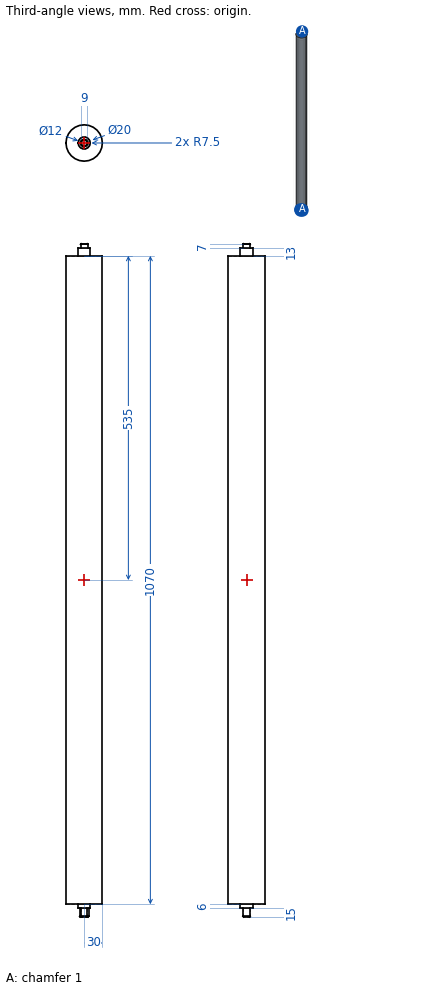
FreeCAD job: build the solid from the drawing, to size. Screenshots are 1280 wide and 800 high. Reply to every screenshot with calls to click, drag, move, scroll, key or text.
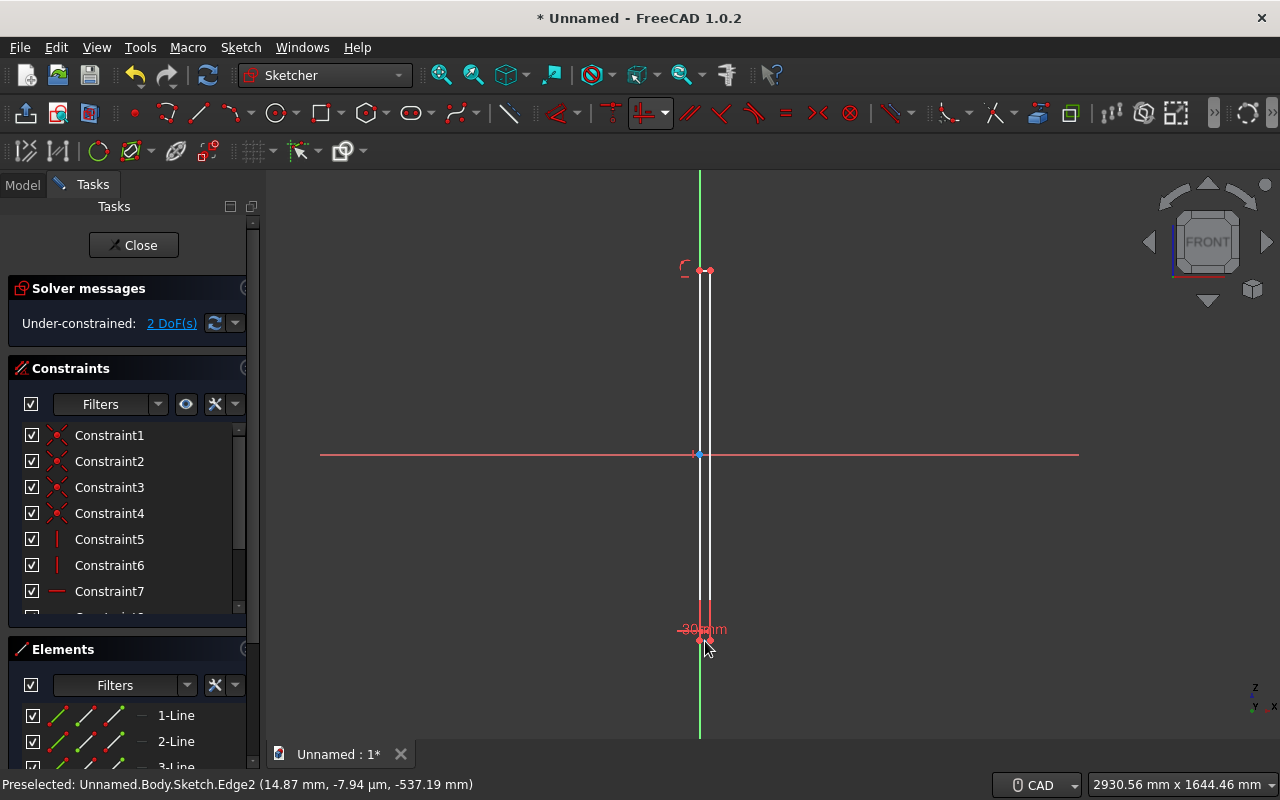
scroll(700, 567, up, 2)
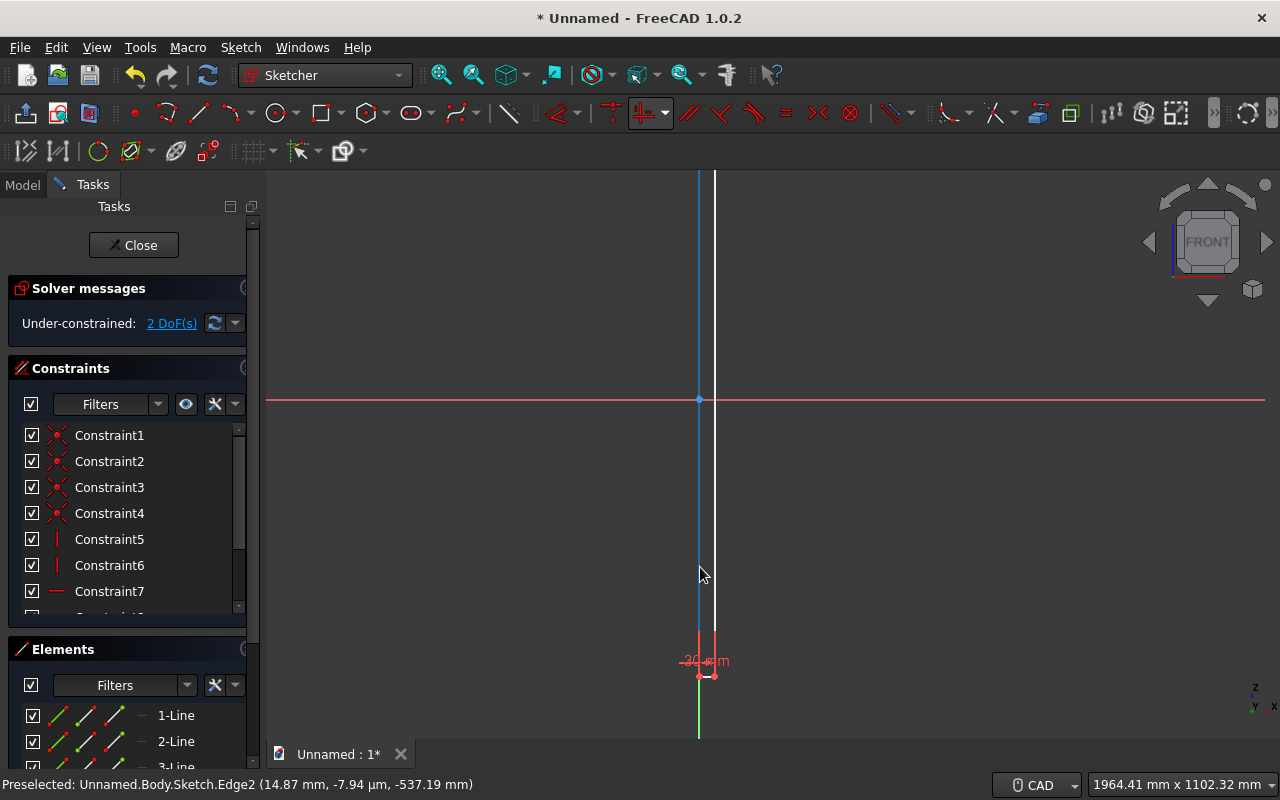
click(699, 566)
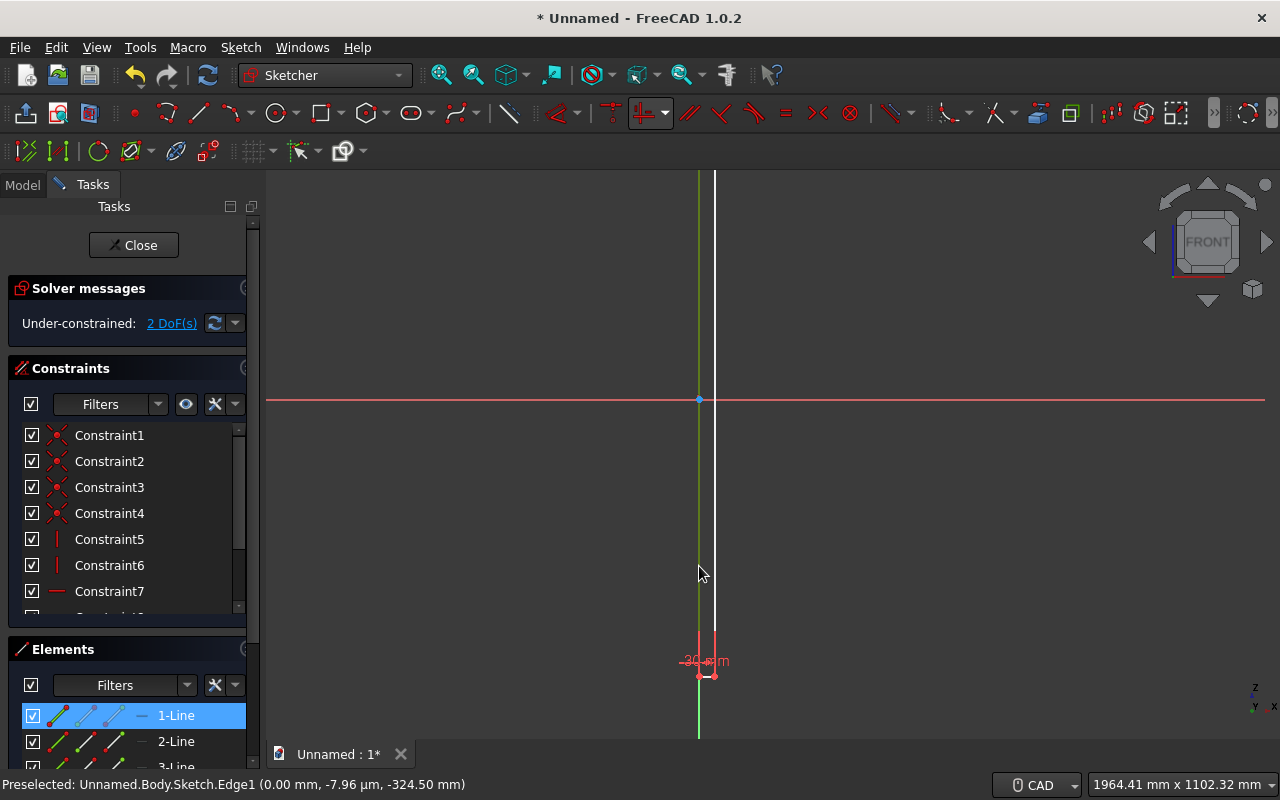
key(i)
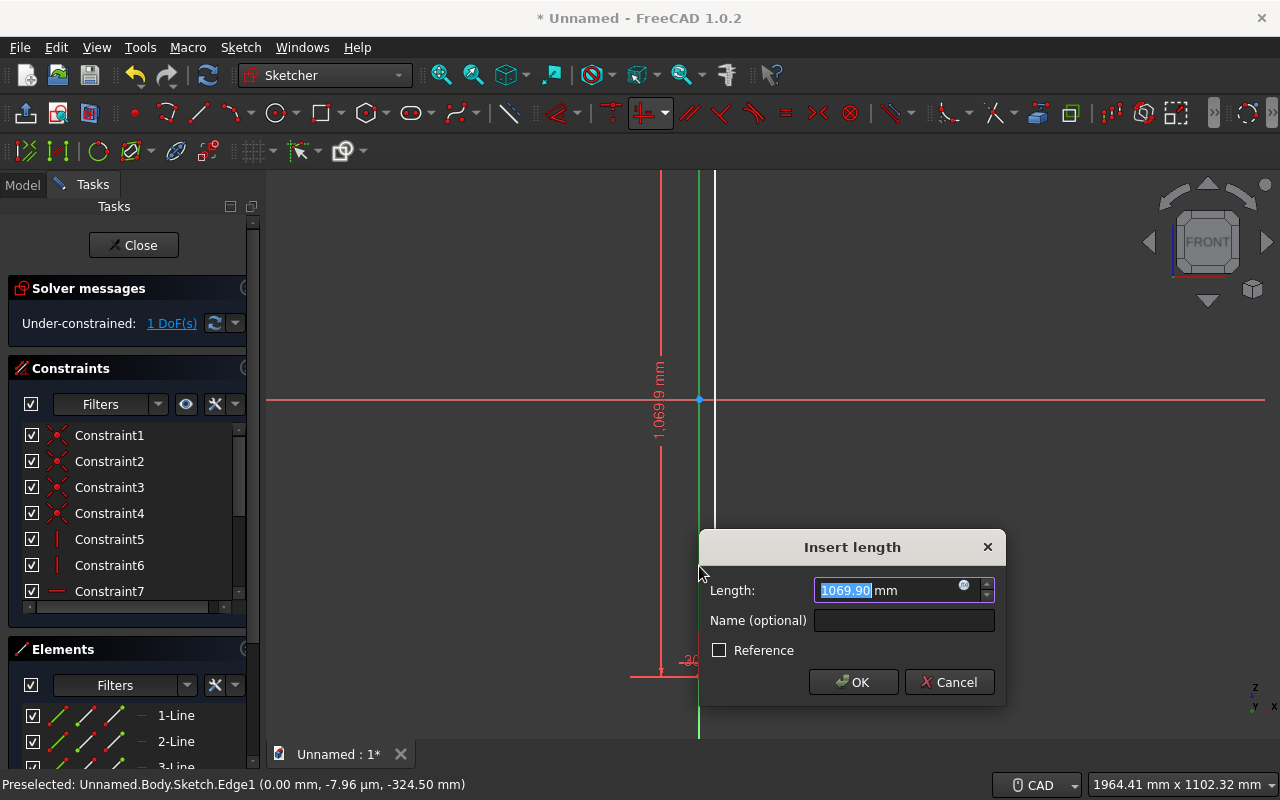
text(1070)
key(Return)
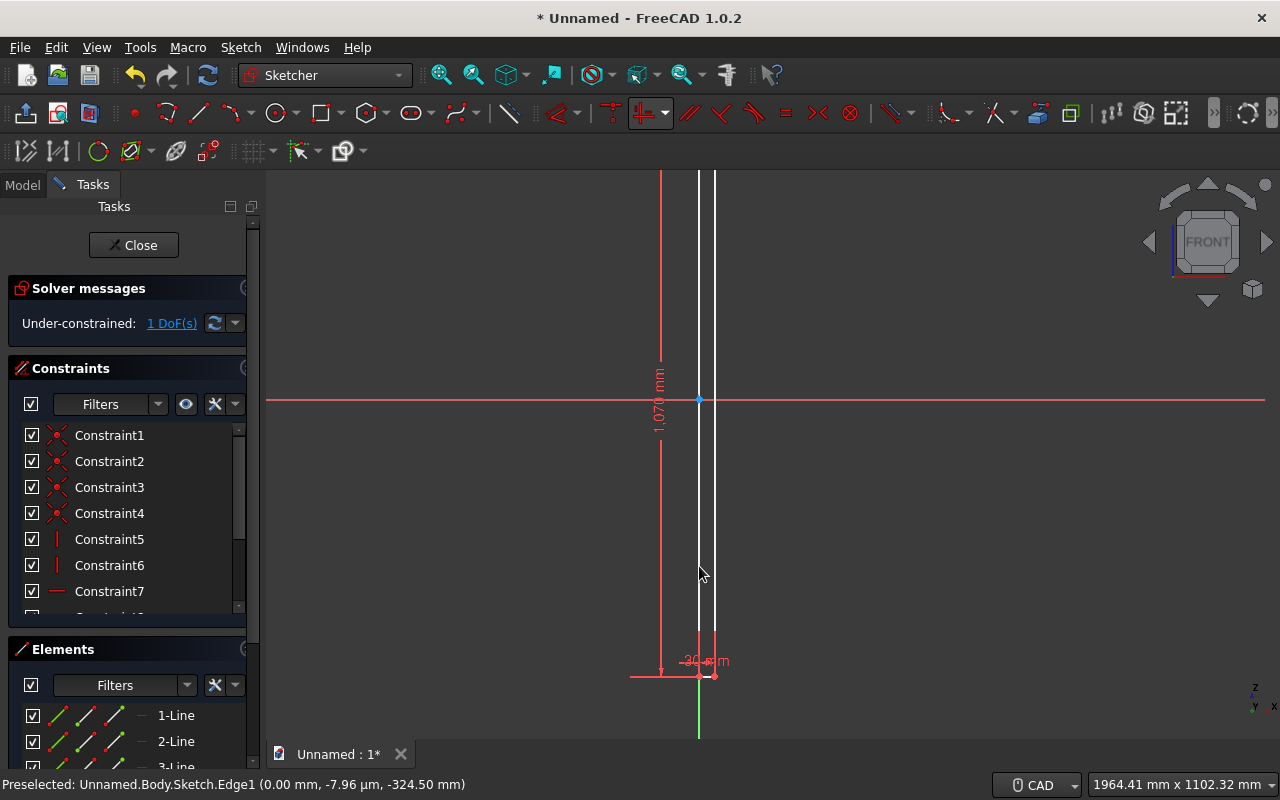
scroll(699, 566, down, 2)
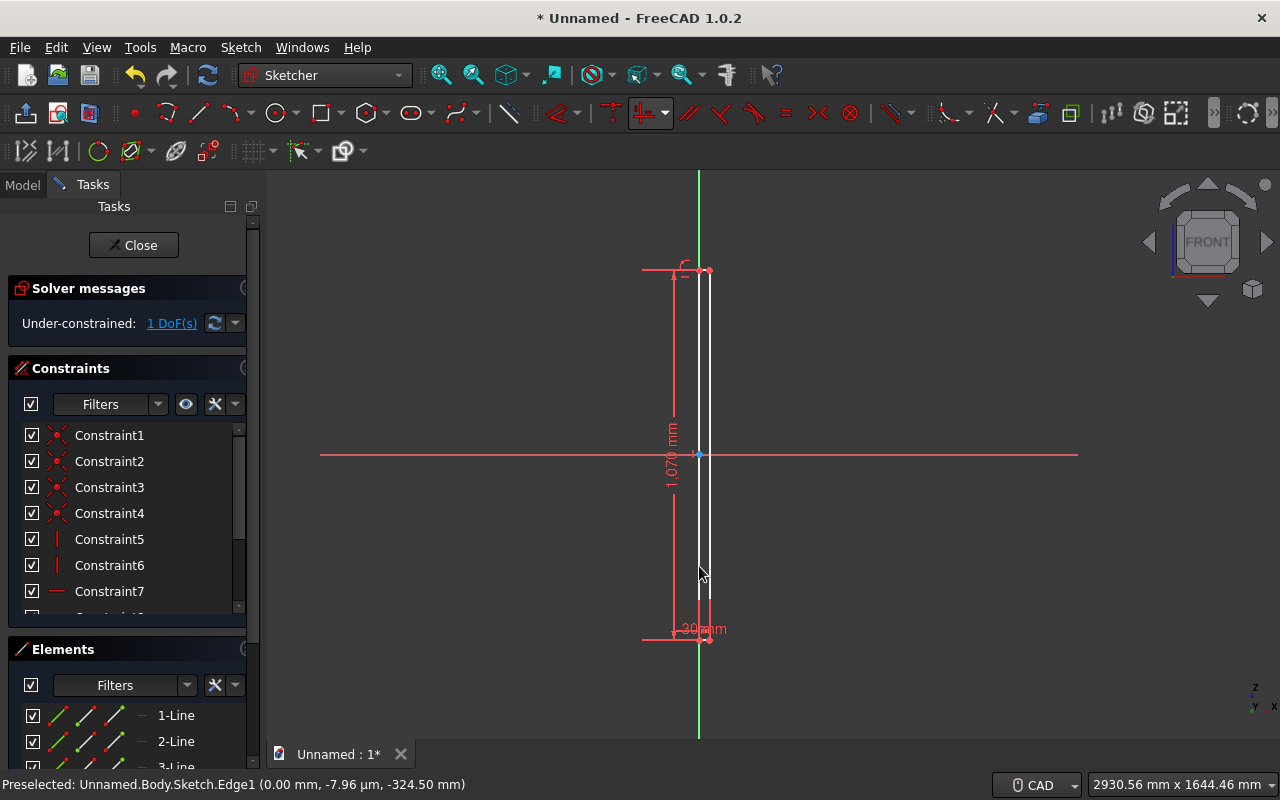
click(699, 270)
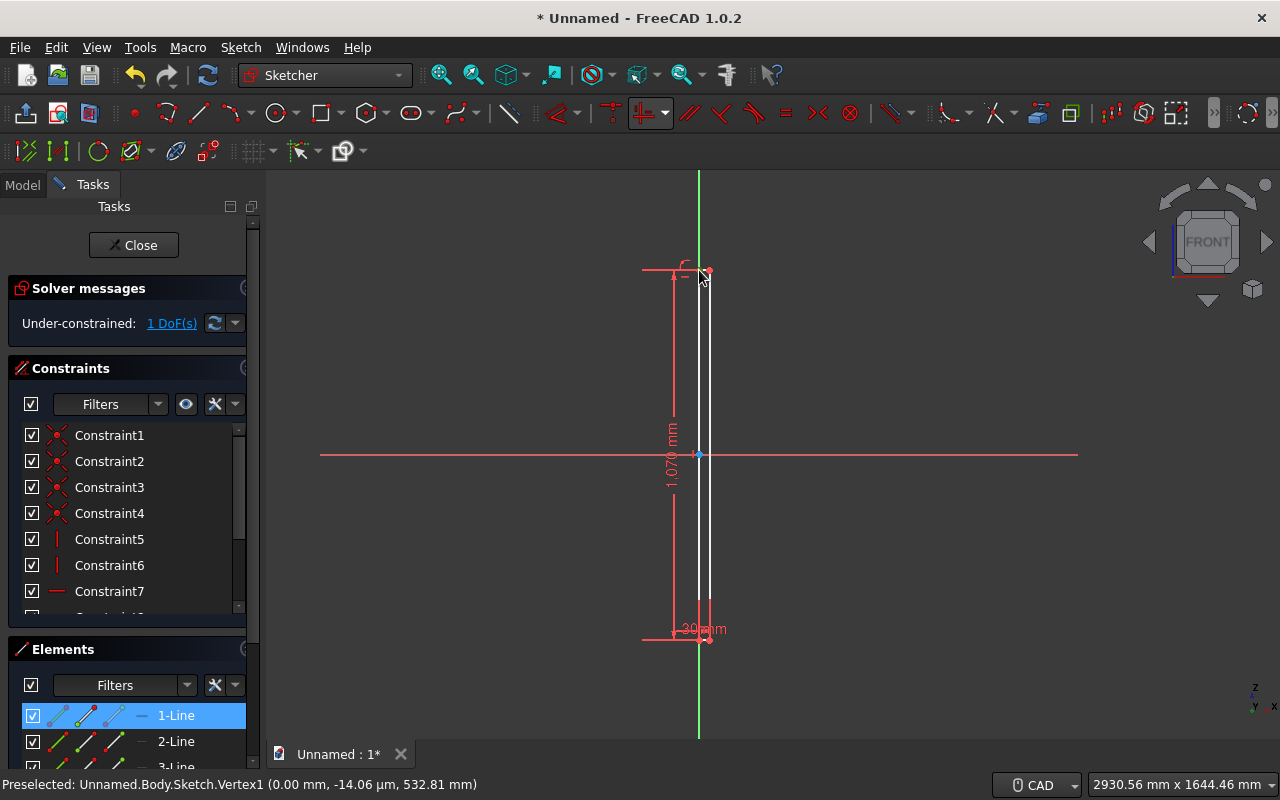
key(i)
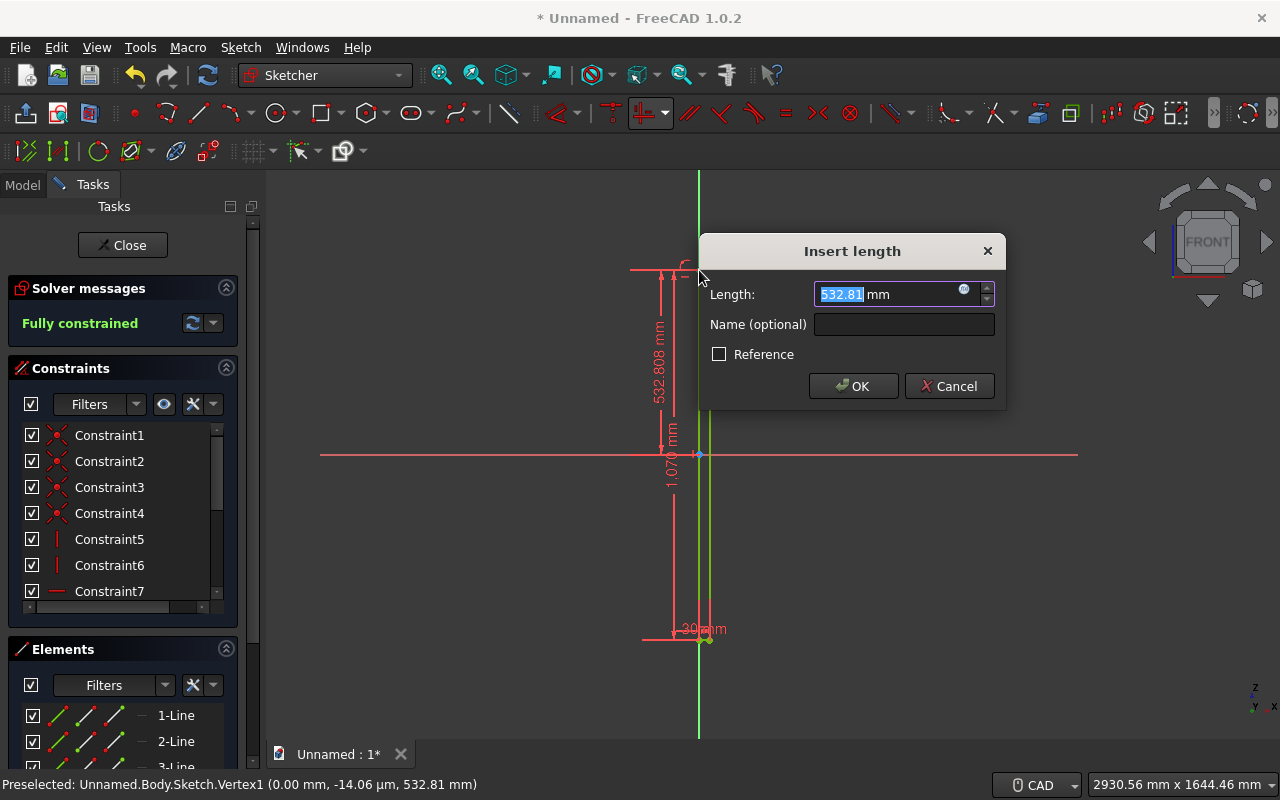
text(535)
key(Return)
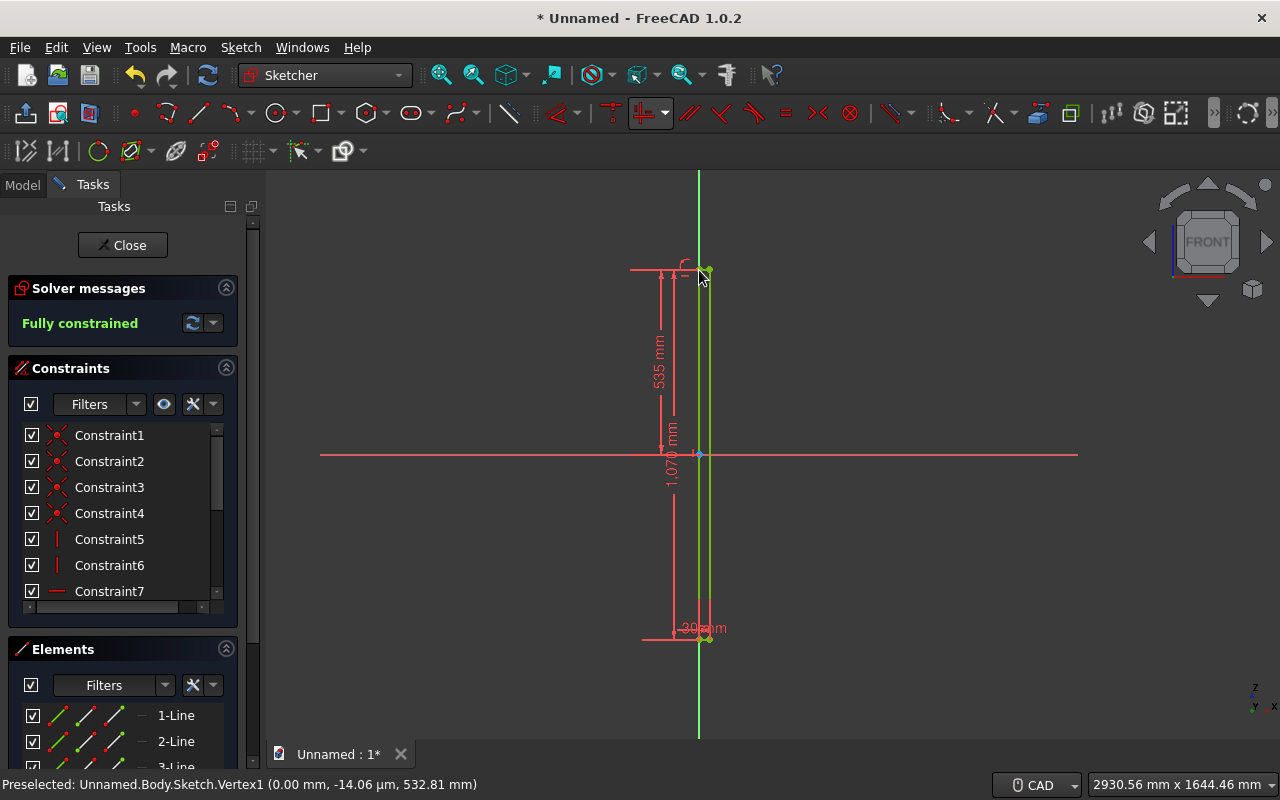
click(123, 245)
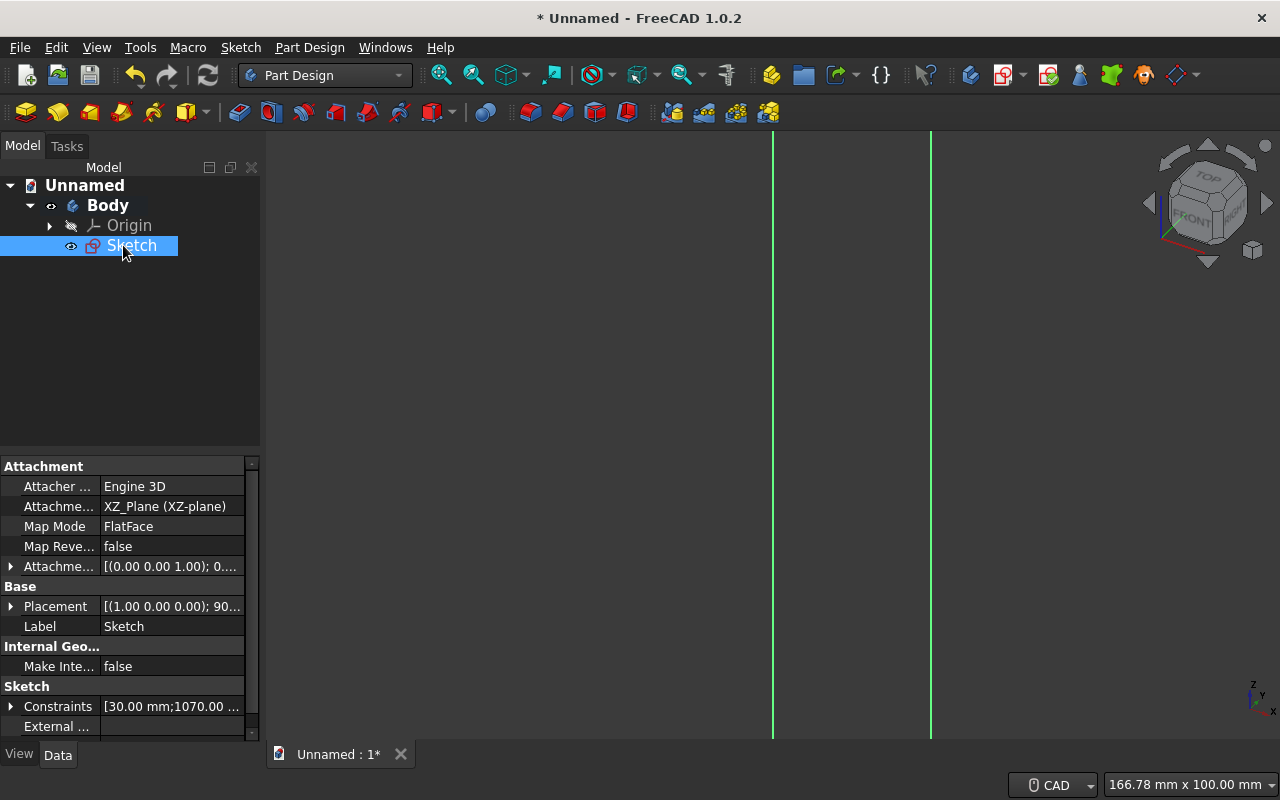
click(58, 112)